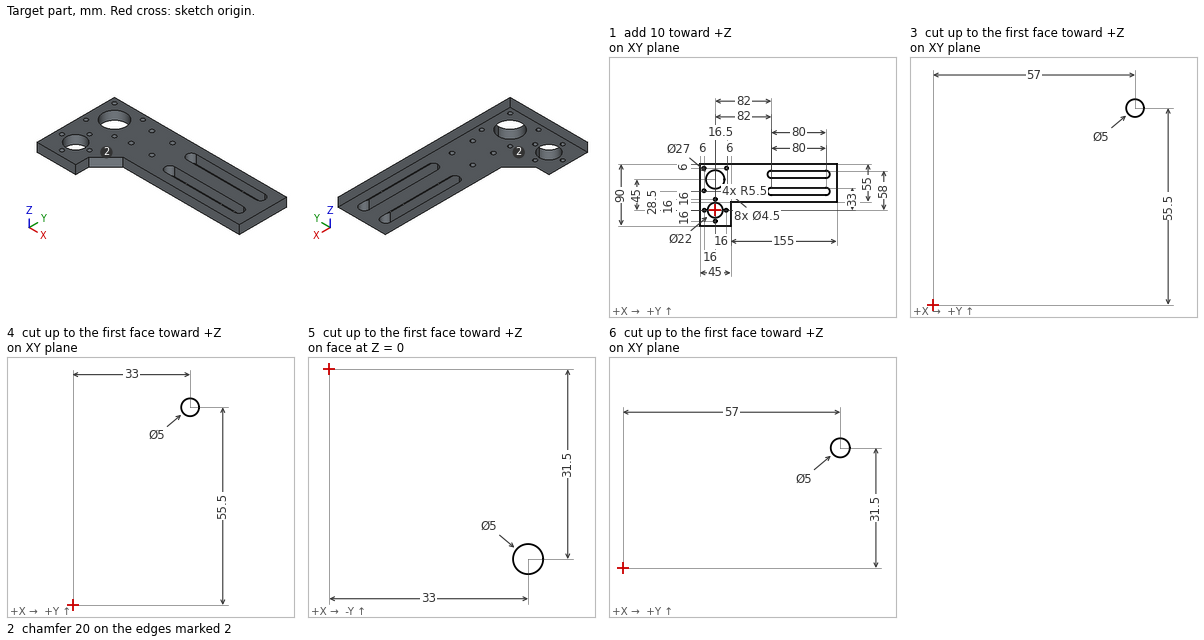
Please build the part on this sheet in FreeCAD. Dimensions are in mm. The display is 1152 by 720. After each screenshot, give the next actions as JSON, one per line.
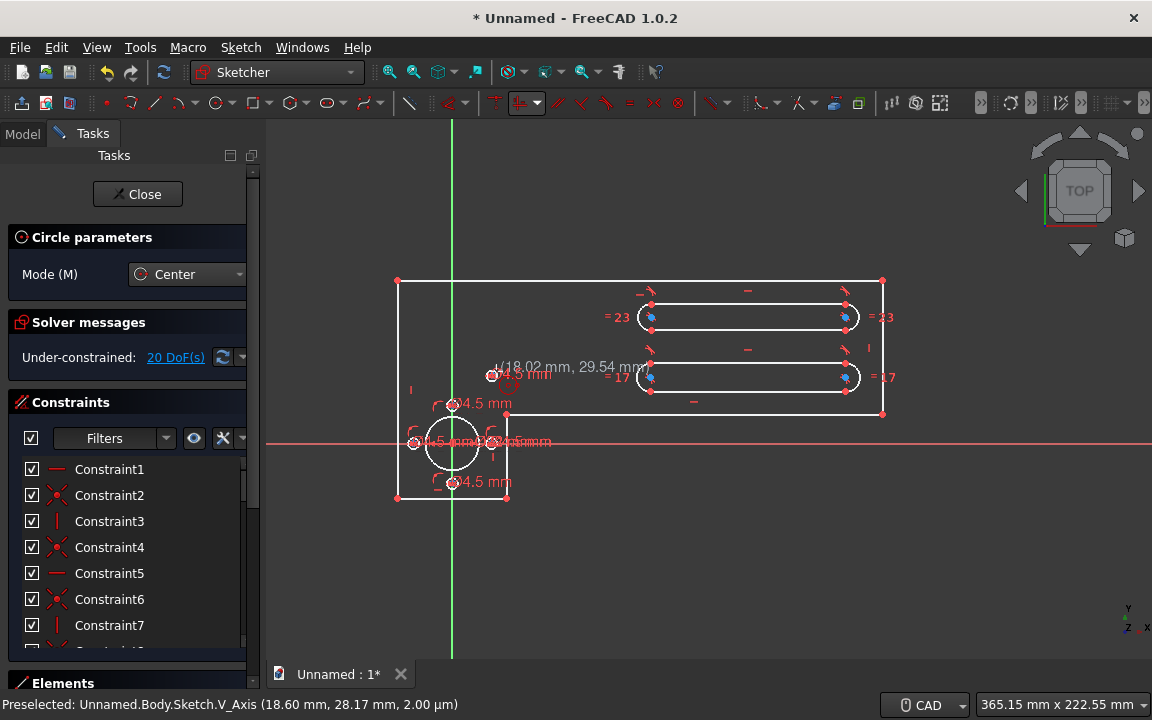
{"action": "scroll", "coordinate": [412, 375], "scroll_direction": "up", "scroll_amount": 8}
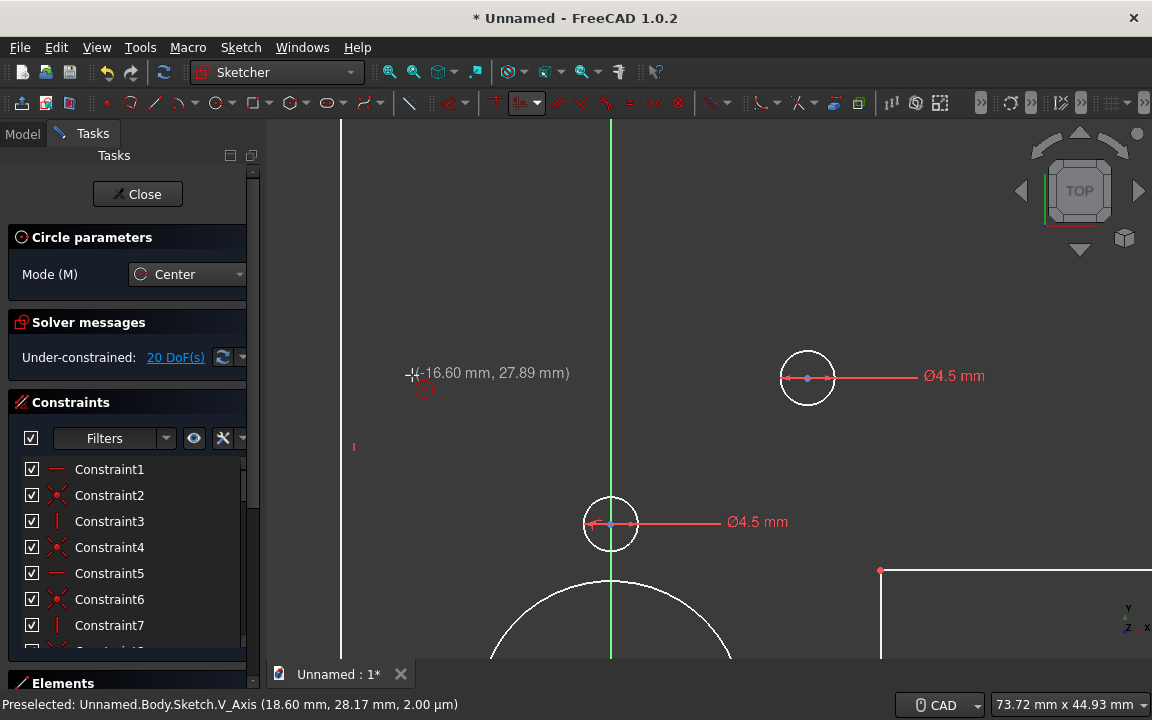
{"action": "scroll", "coordinate": [412, 375], "scroll_direction": "down", "scroll_amount": 8}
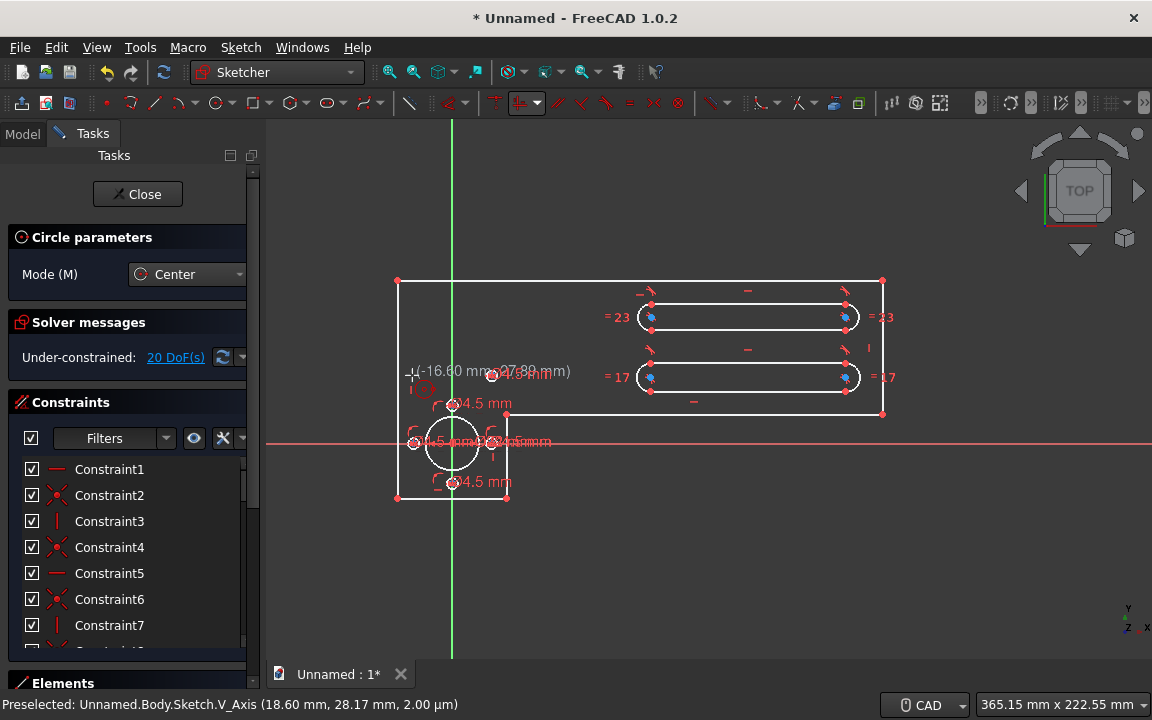
{"action": "left_click", "coordinate": [412, 375]}
{"action": "mouse_move", "coordinate": [416, 371]}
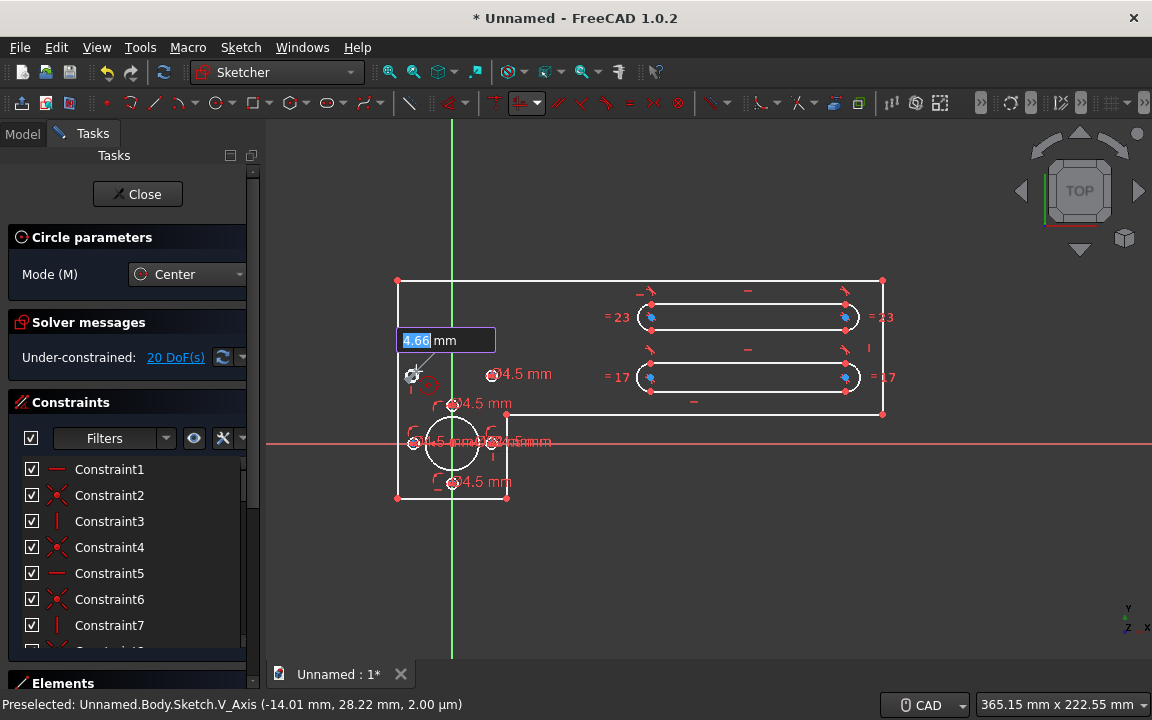
{"action": "type", "text": "4.5"}
{"action": "key", "text": "Return"}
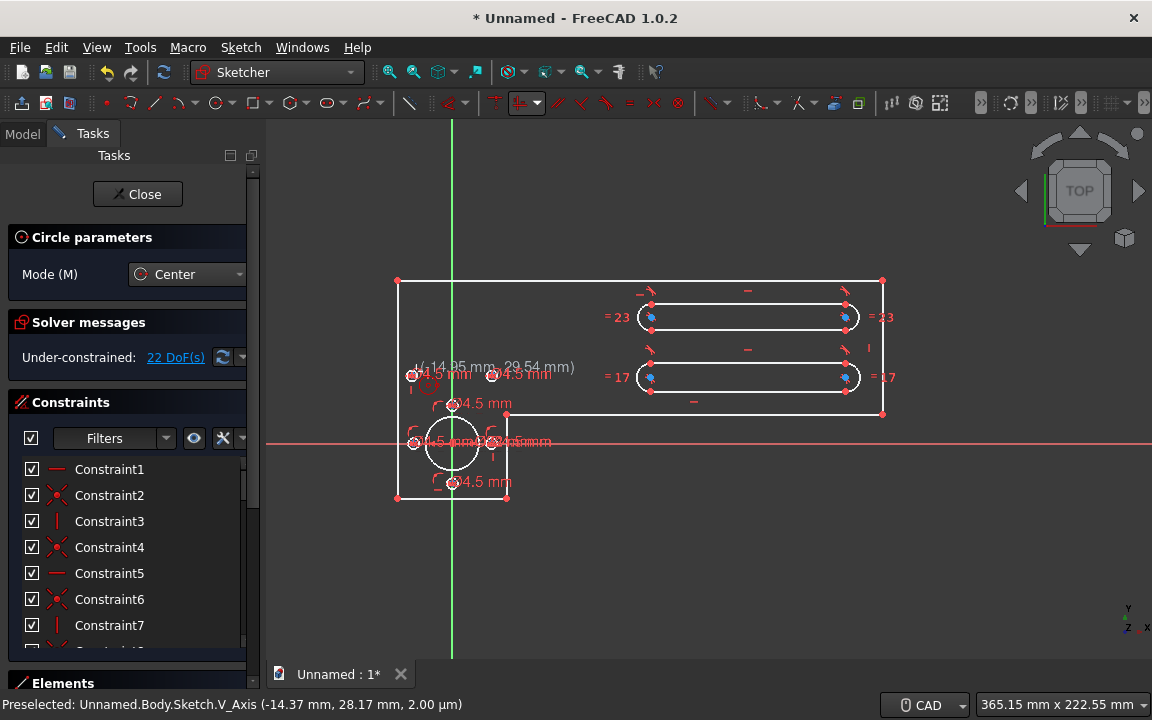
{"action": "left_click", "coordinate": [452, 334]}
{"action": "mouse_move", "coordinate": [475, 311]}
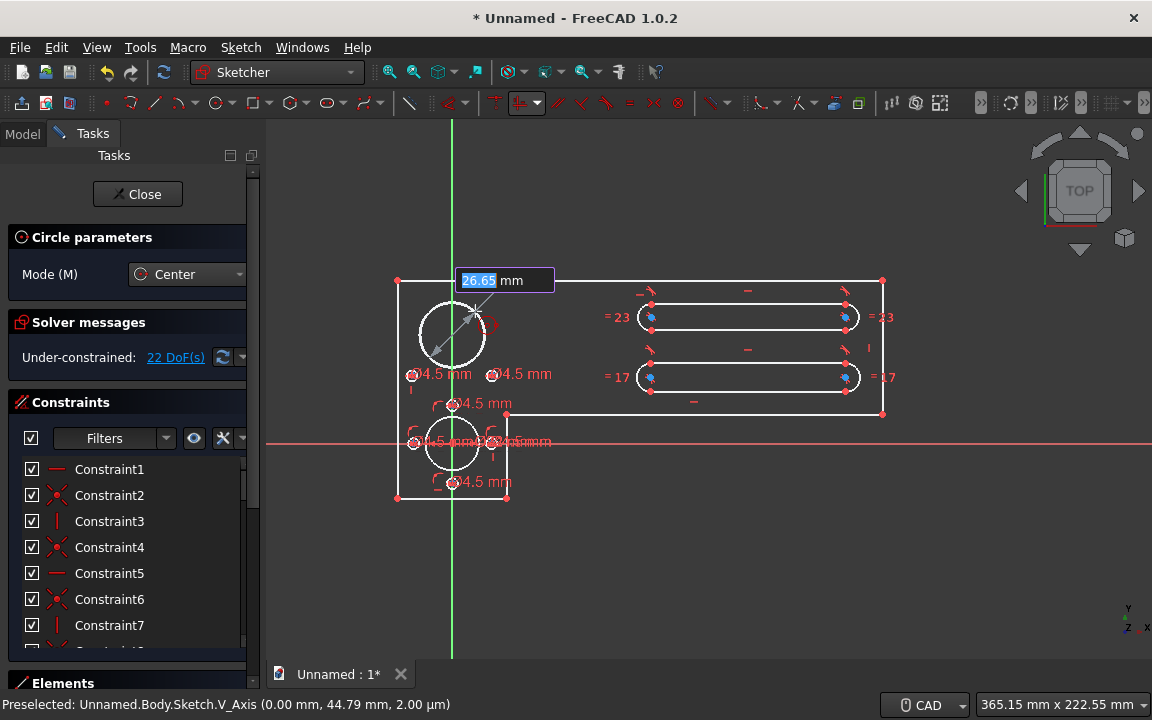
{"action": "type", "text": "27"}
{"action": "key", "text": "Return"}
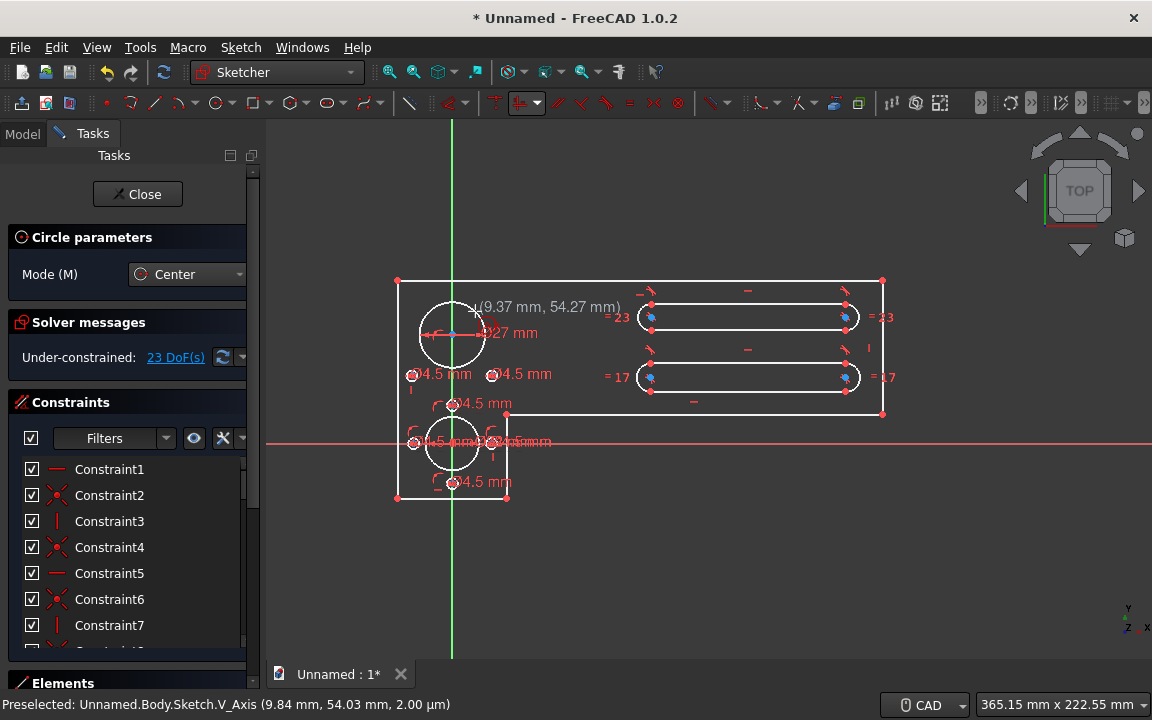
{"action": "scroll", "coordinate": [492, 294], "scroll_direction": "up", "scroll_amount": 8}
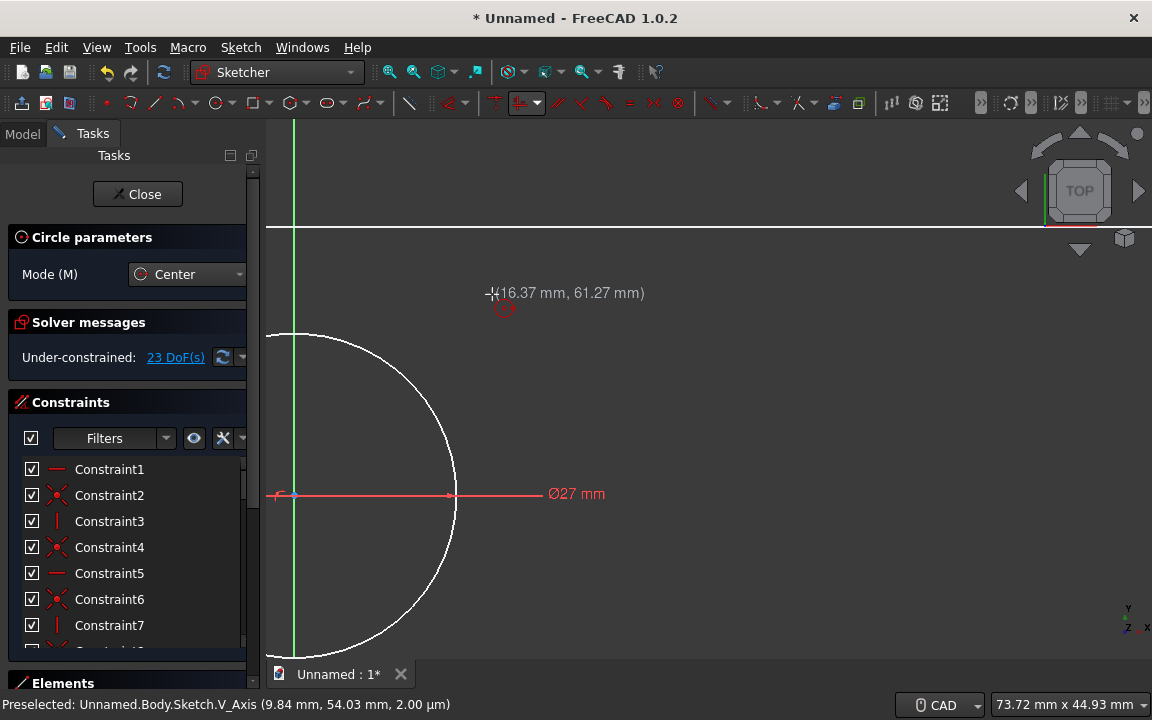
{"action": "scroll", "coordinate": [492, 294], "scroll_direction": "down", "scroll_amount": 8}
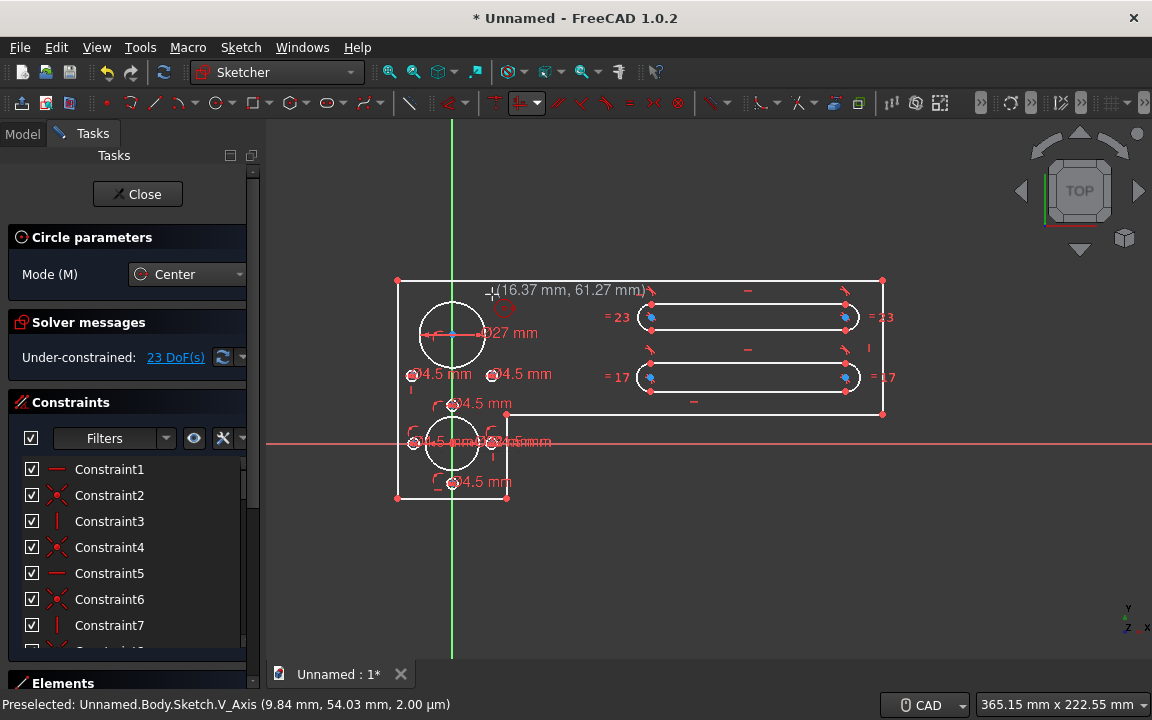
{"action": "left_click", "coordinate": [492, 294]}
{"action": "mouse_move", "coordinate": [496, 298]}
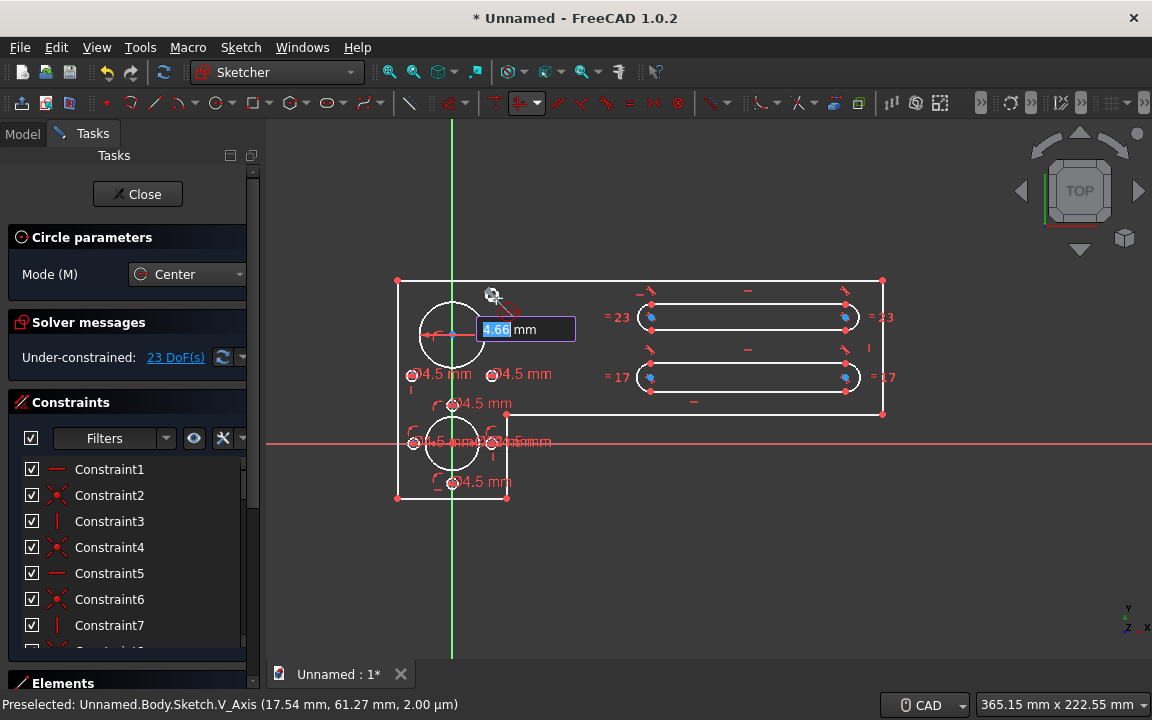
{"action": "type", "text": "4.5"}
{"action": "key", "text": "Return"}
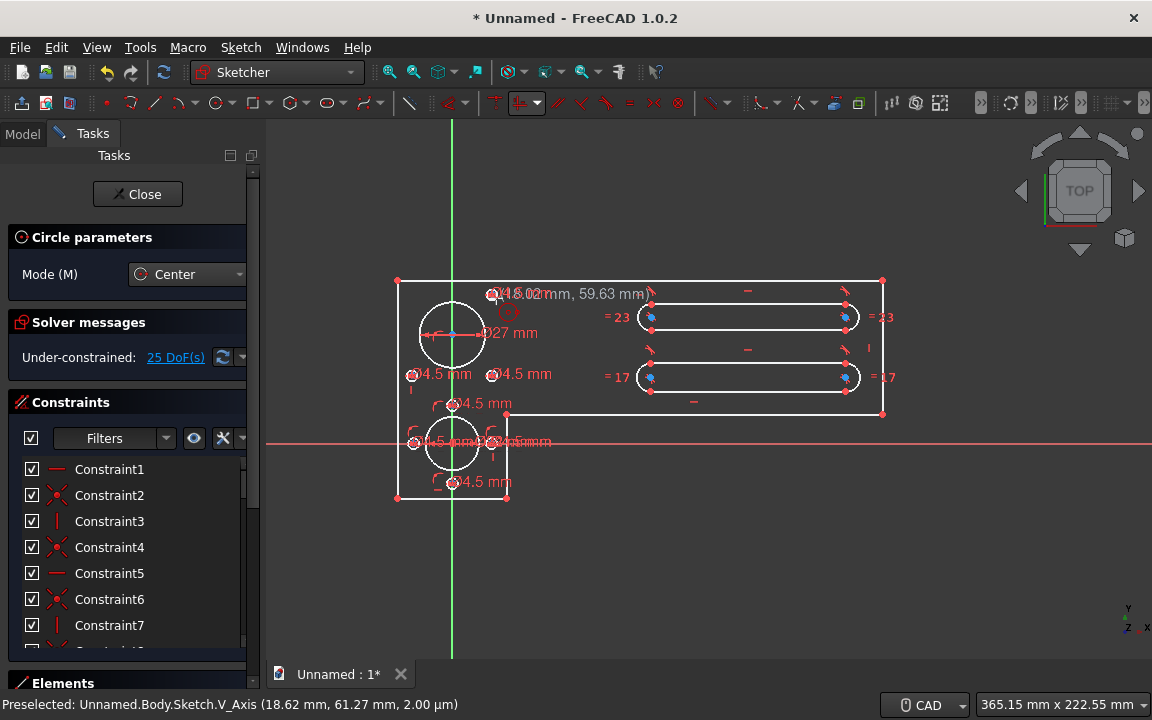
{"action": "scroll", "coordinate": [412, 294], "scroll_direction": "up", "scroll_amount": 8}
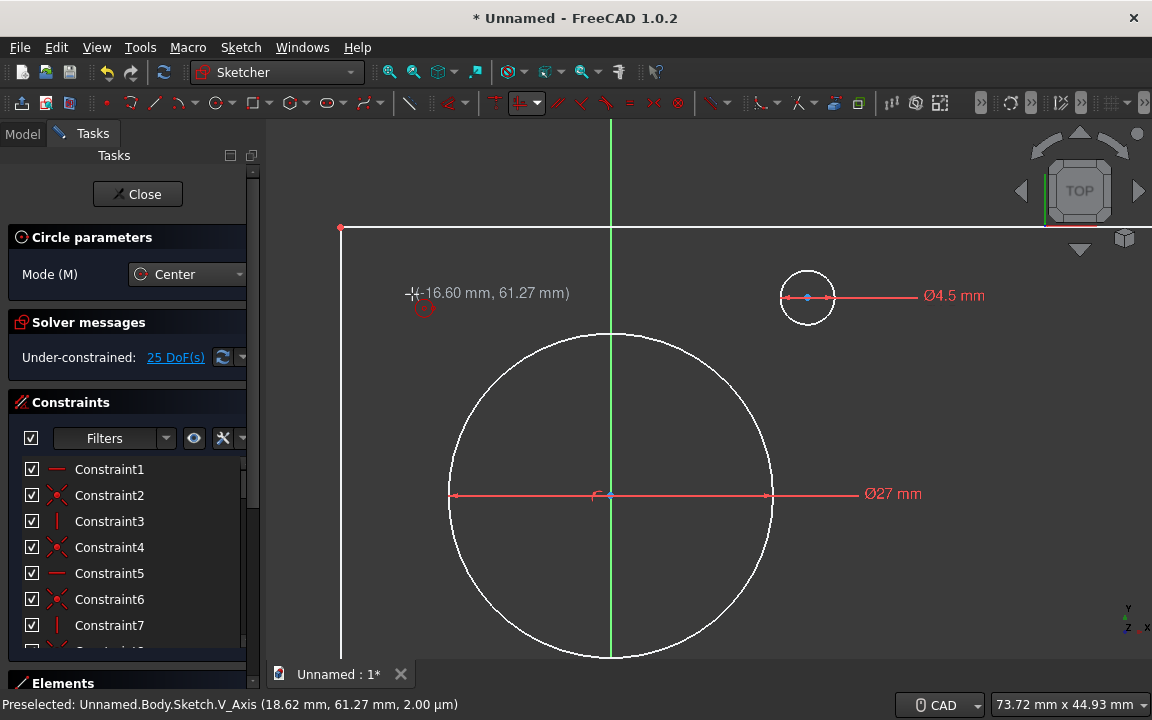
{"action": "scroll", "coordinate": [412, 294], "scroll_direction": "down", "scroll_amount": 8}